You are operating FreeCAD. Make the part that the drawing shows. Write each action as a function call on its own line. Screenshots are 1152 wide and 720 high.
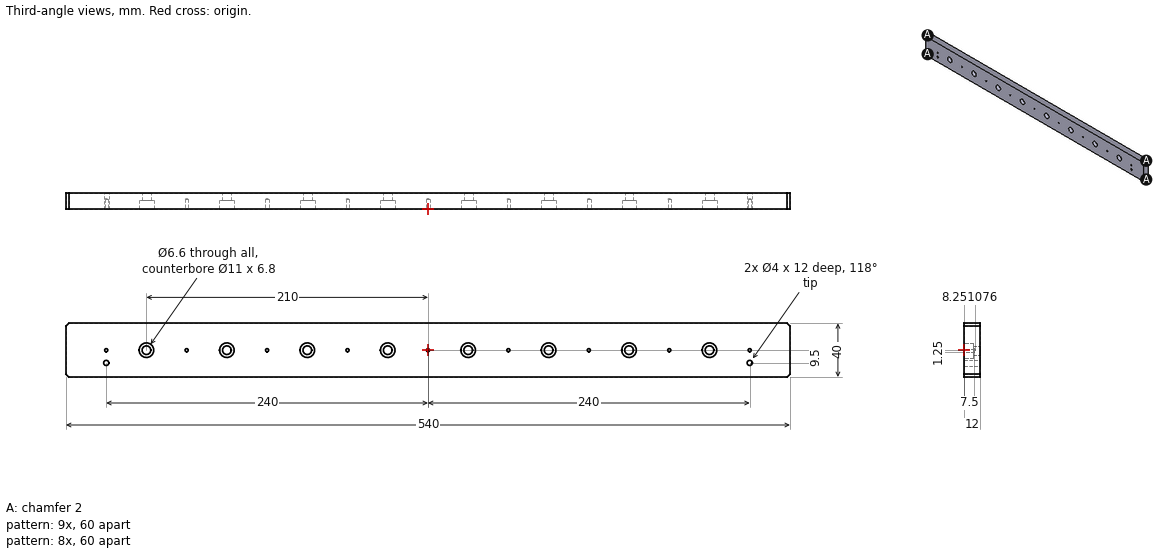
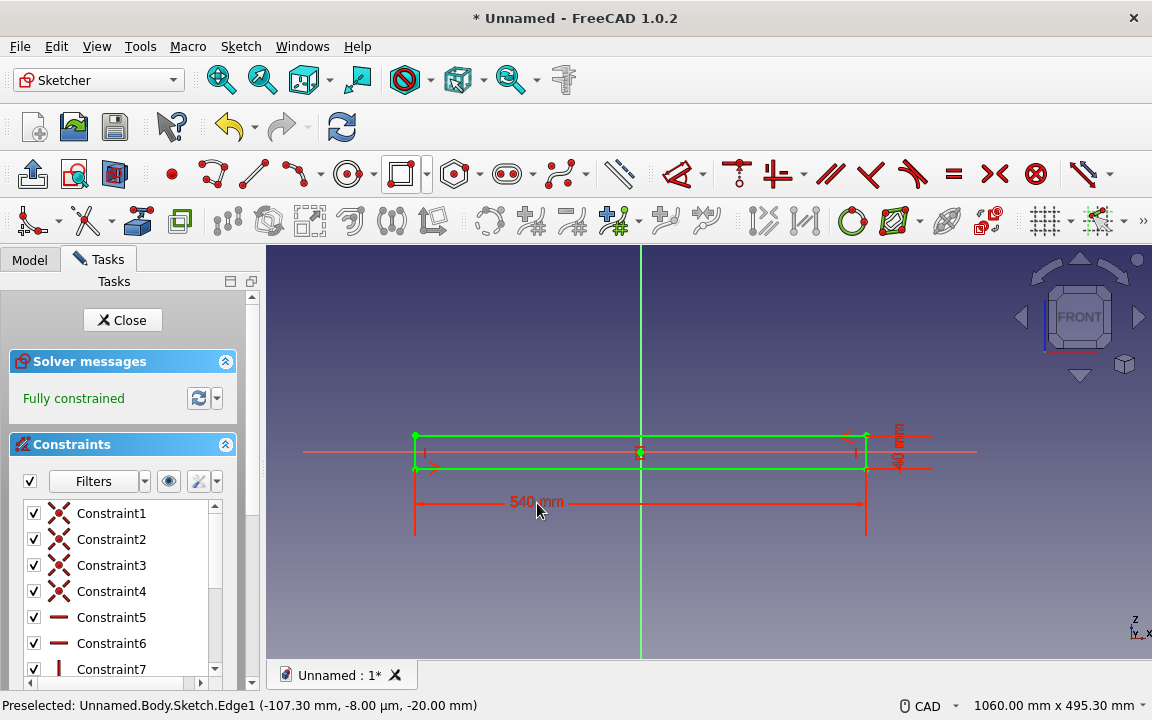
click(123, 320)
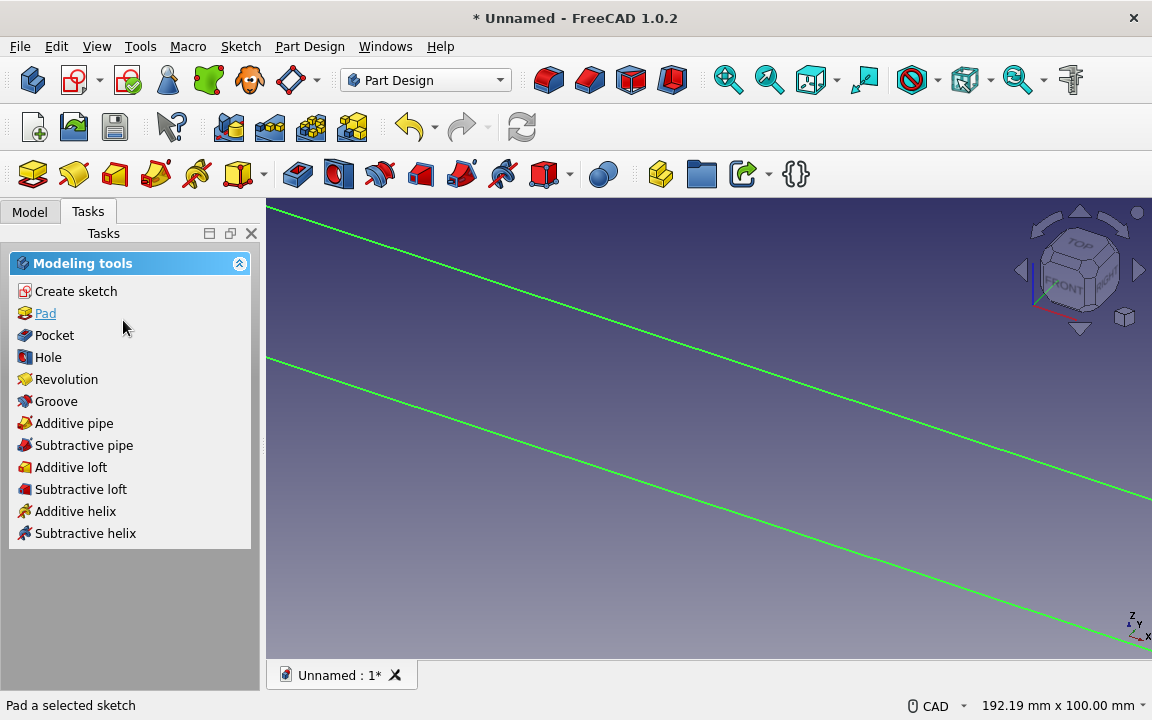
click(33, 174)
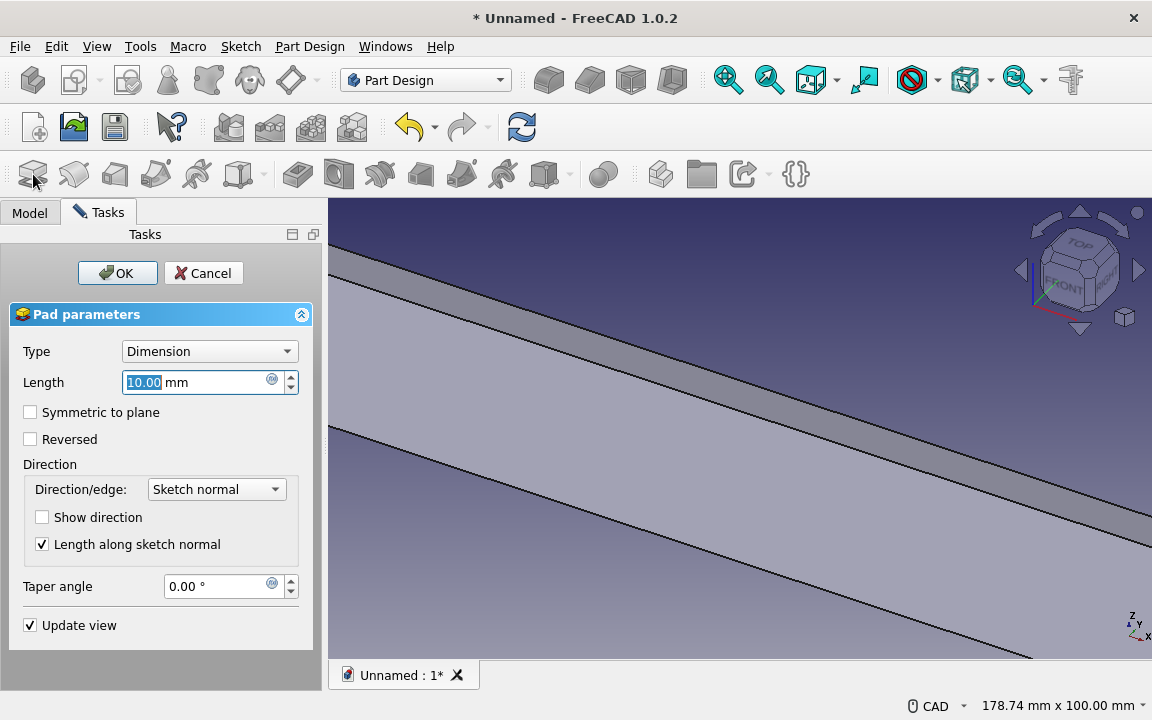
text(12)
key(Tab)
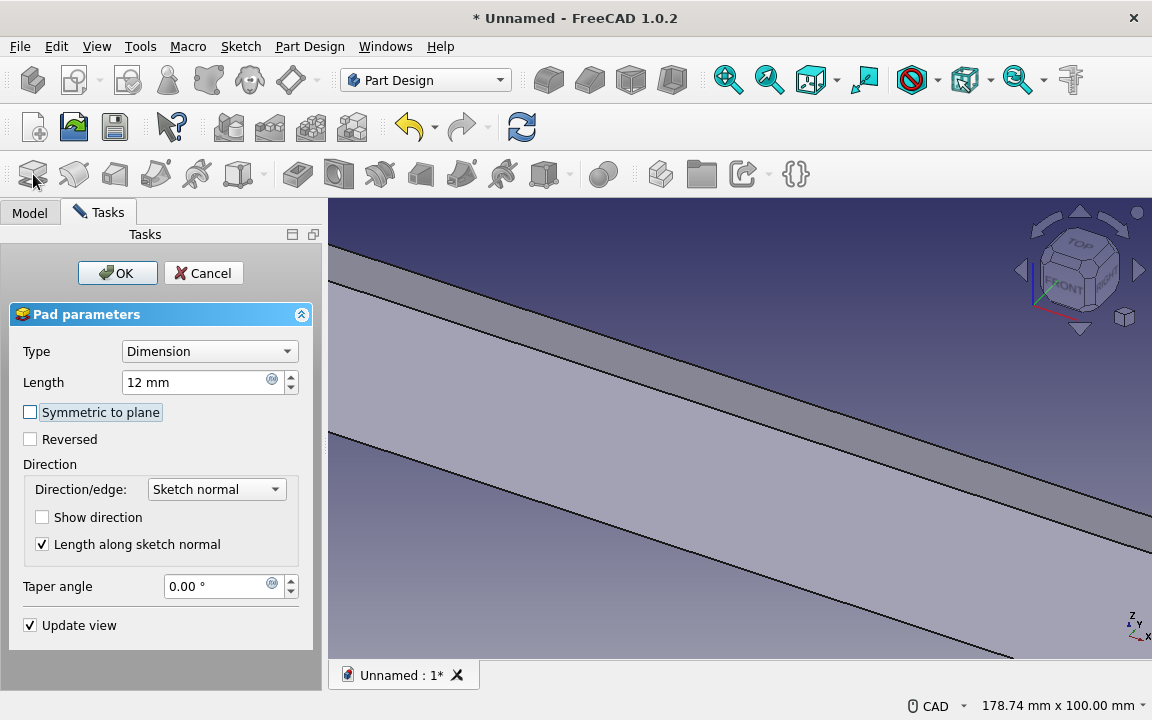
click(31, 439)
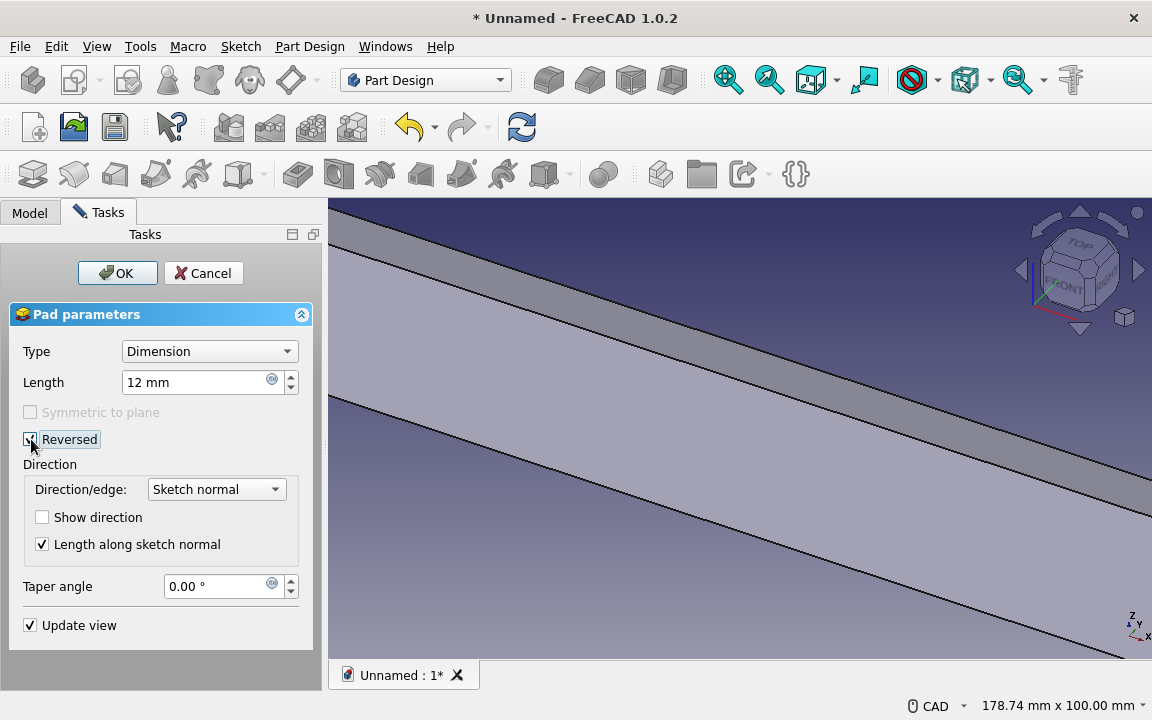
click(118, 273)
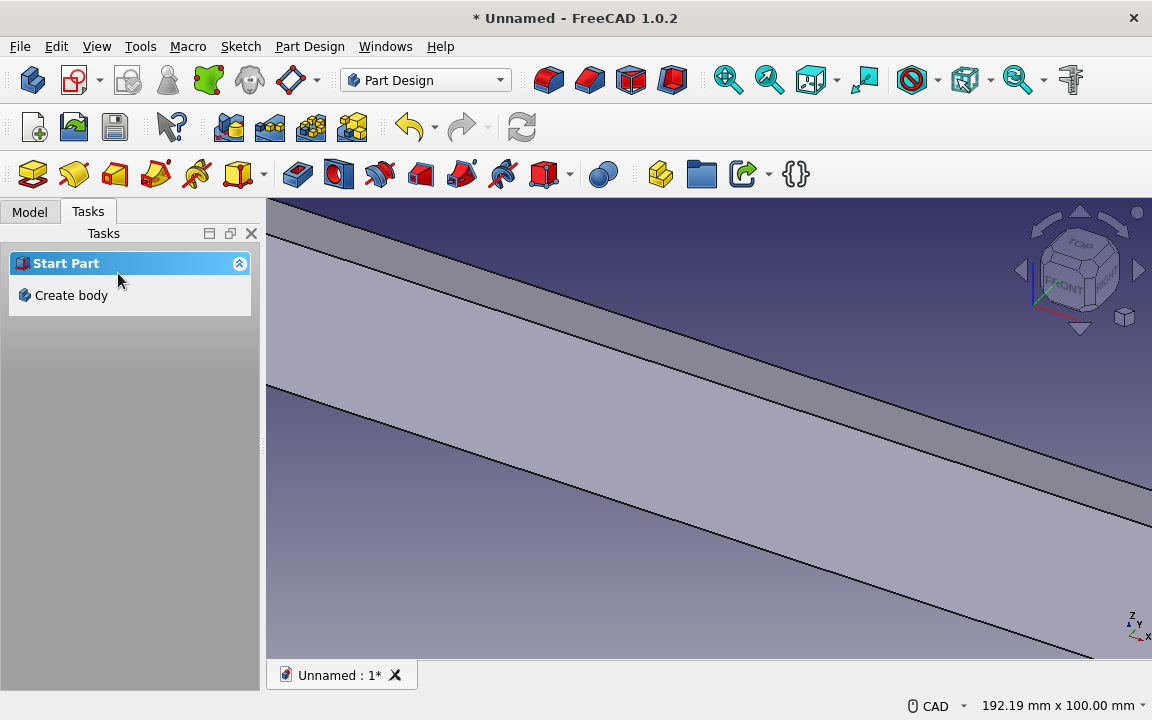
key(v)
key(f)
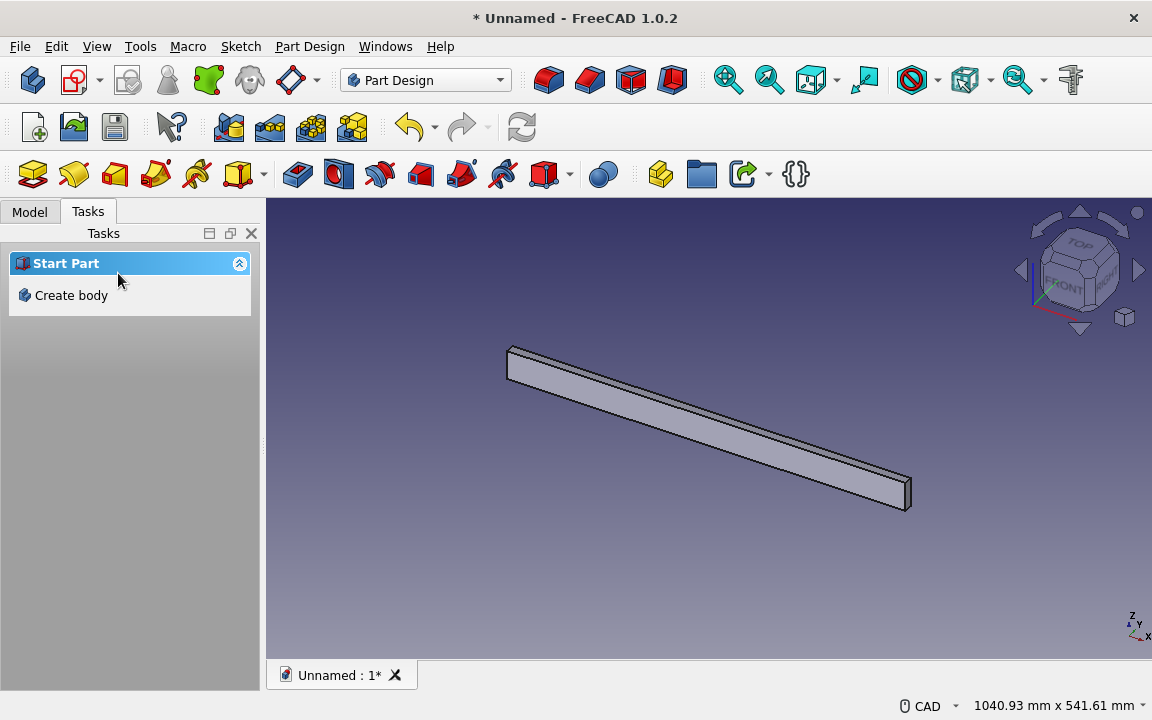
scroll(908, 479, up, 7)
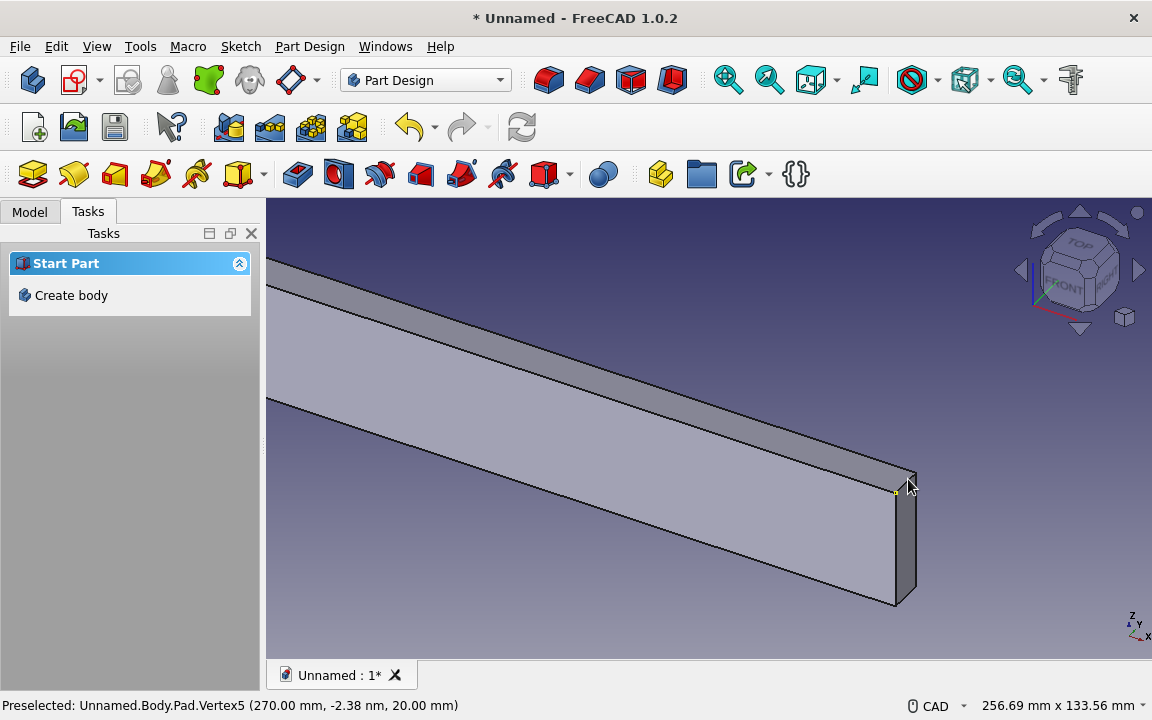
click(906, 482)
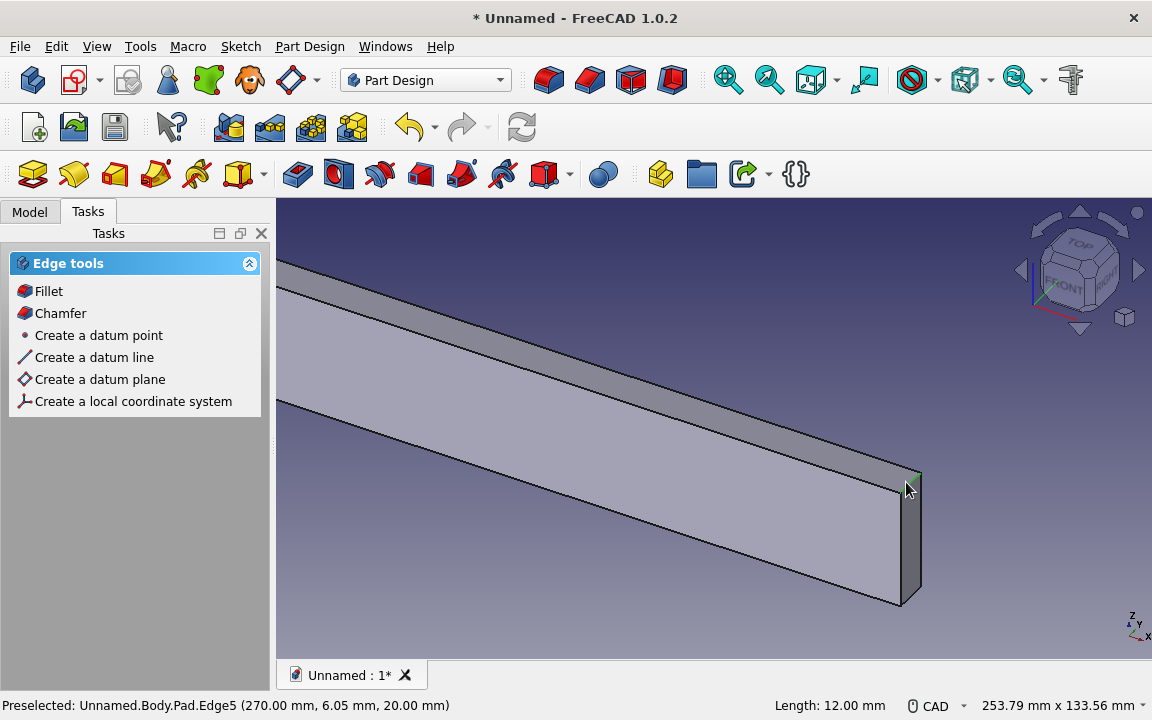
click(729, 80)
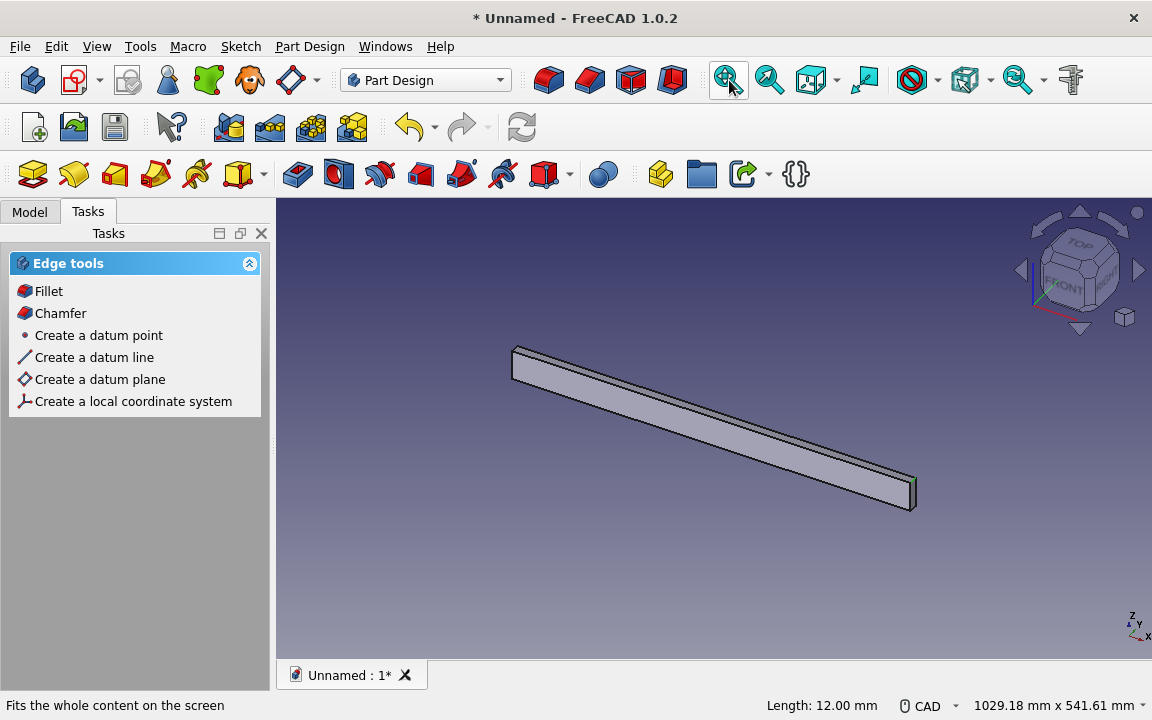
key(0)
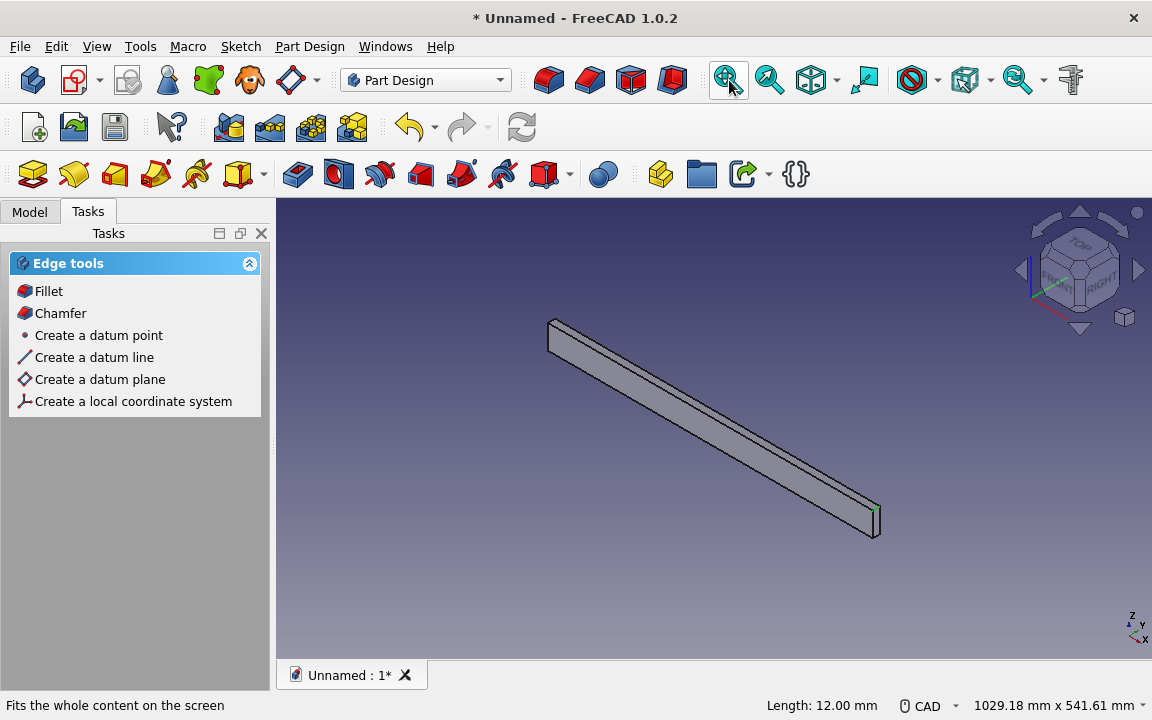
scroll(551, 320, up, 7)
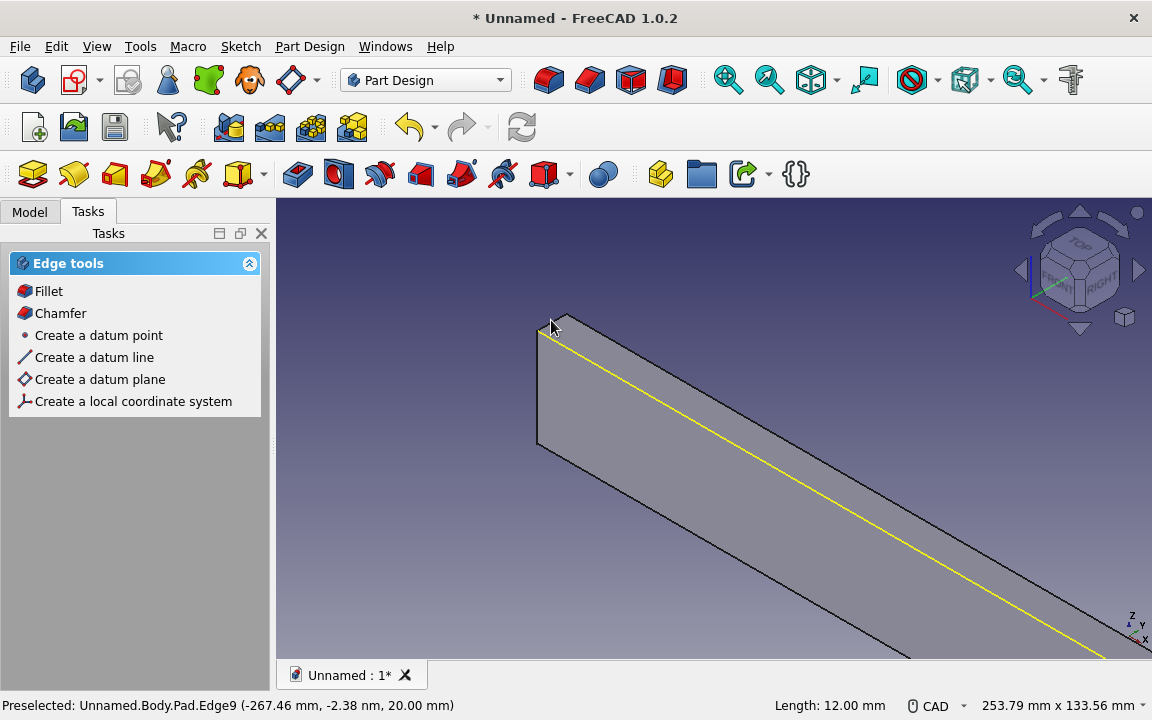
click(729, 80)